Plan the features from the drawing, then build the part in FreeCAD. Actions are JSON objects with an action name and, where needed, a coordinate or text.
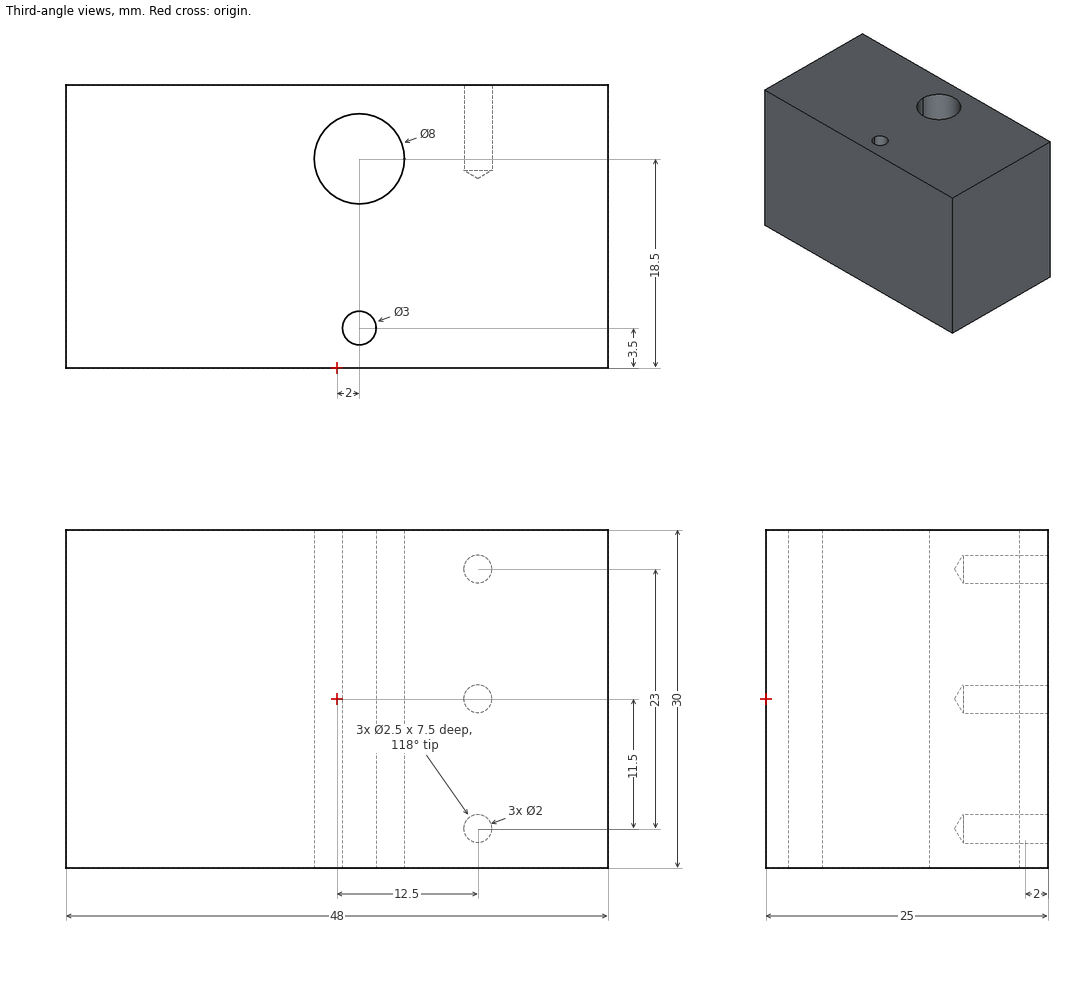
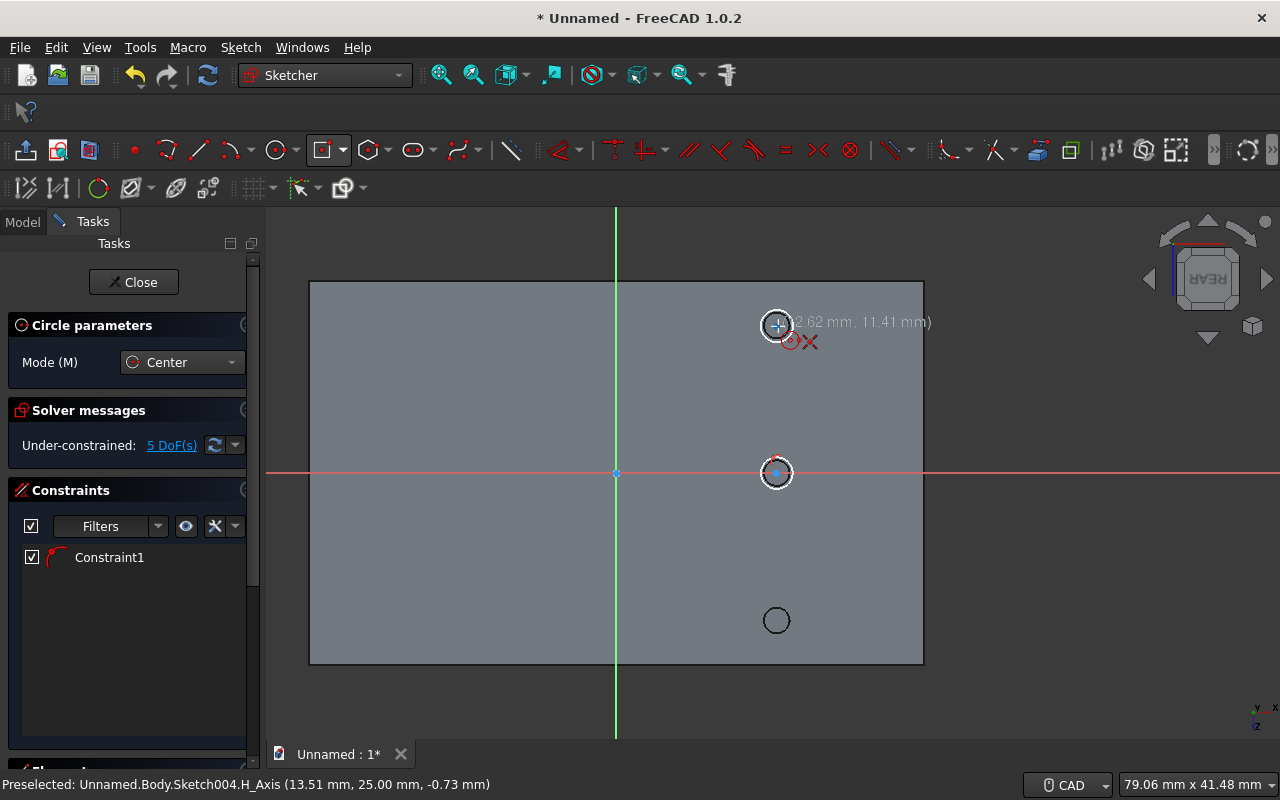
{"action": "scroll", "coordinate": [777, 621], "scroll_direction": "up", "scroll_amount": 2}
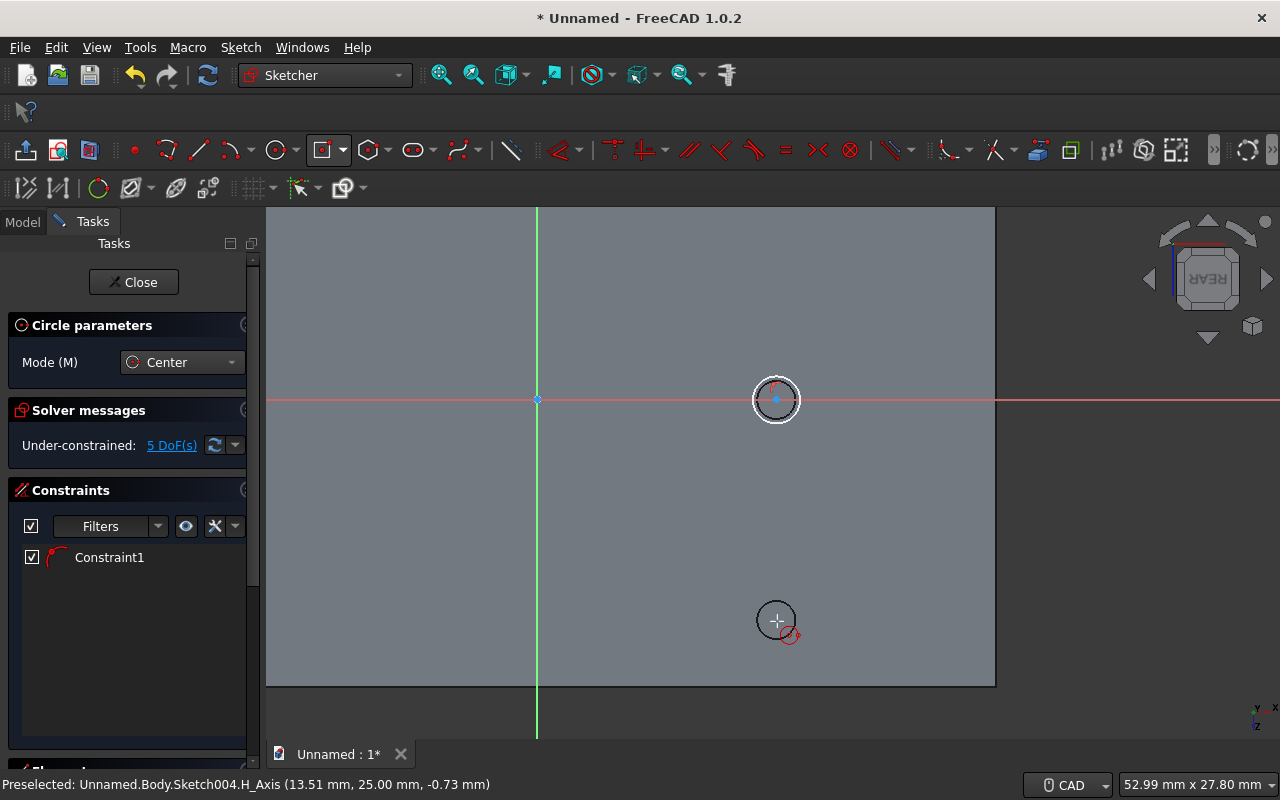
{"action": "left_click", "coordinate": [776, 620]}
{"action": "left_click", "coordinate": [793, 603]}
{"action": "key", "text": "Escape"}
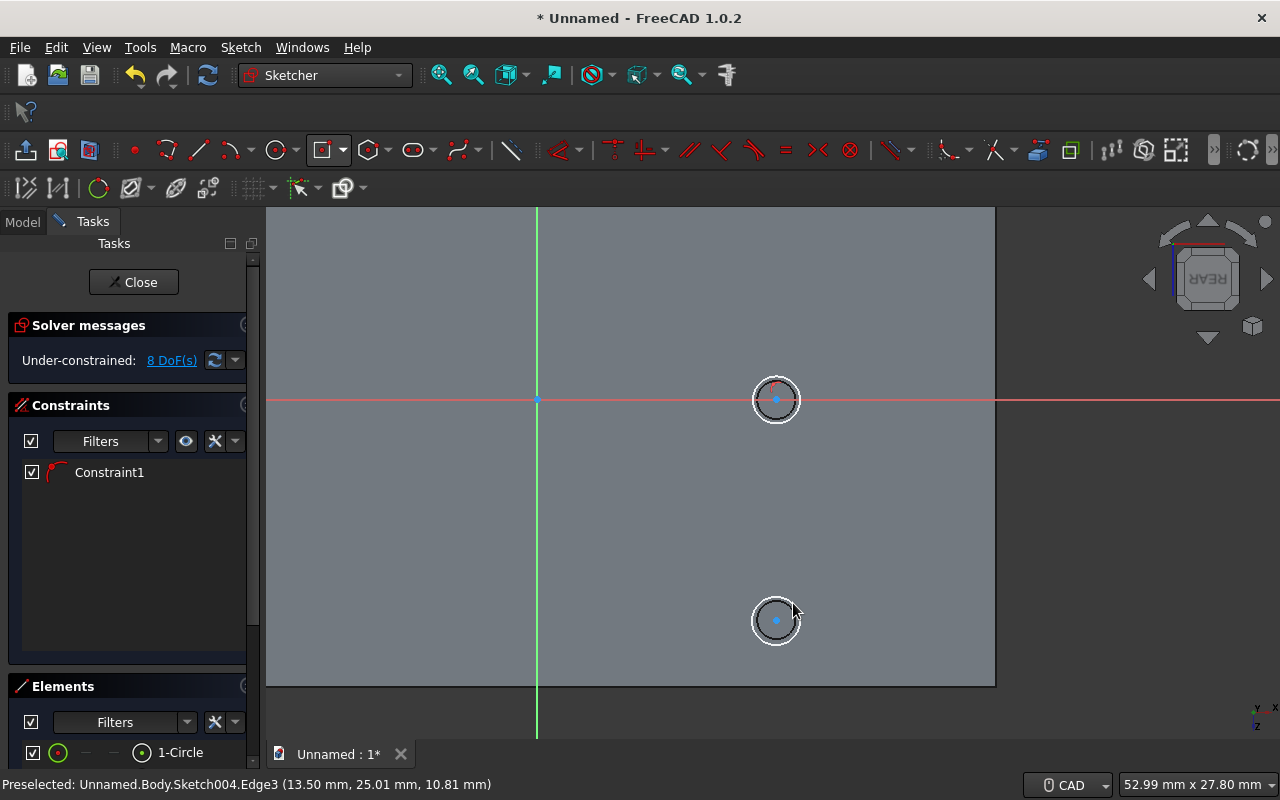
{"action": "scroll", "coordinate": [777, 622], "scroll_direction": "down", "scroll_amount": 2}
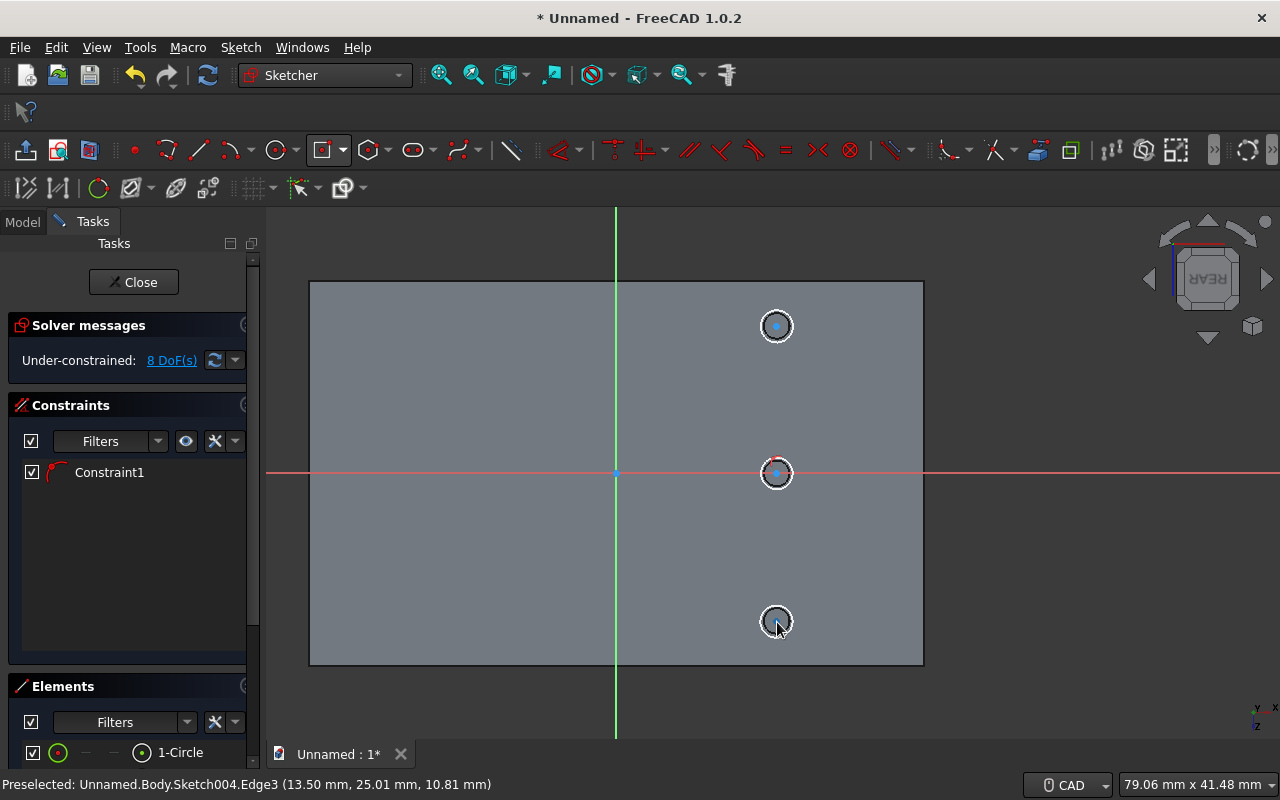
{"action": "left_click", "coordinate": [788, 315]}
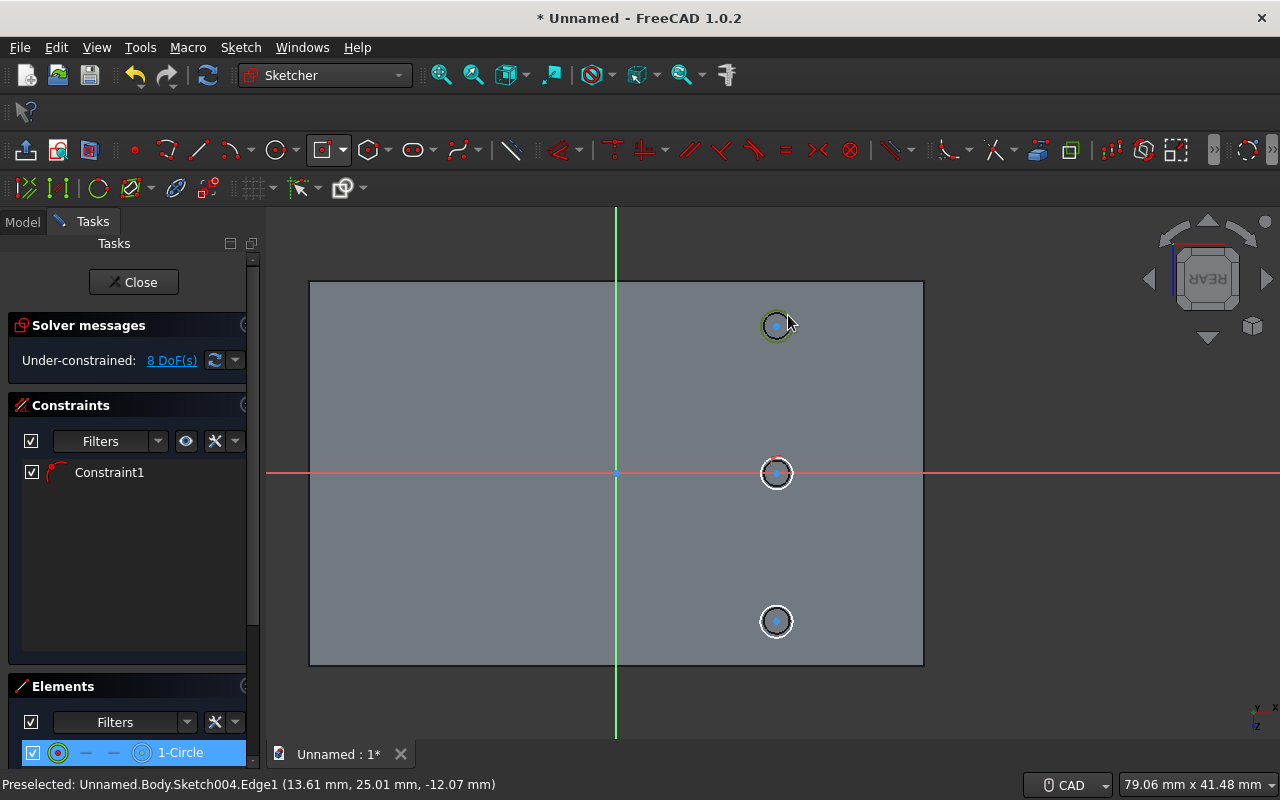
{"action": "scroll", "coordinate": [788, 462], "scroll_direction": "up", "scroll_amount": 2}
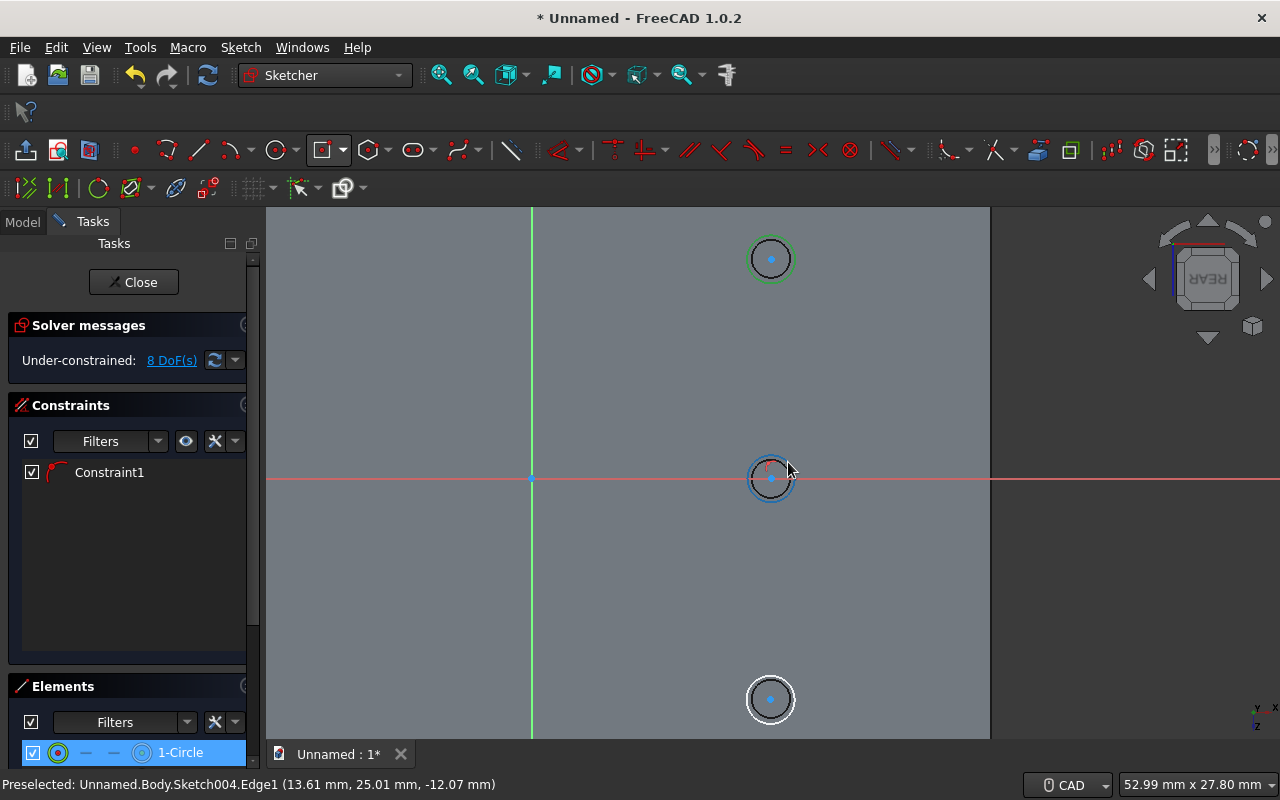
{"action": "left_click", "coordinate": [788, 462]}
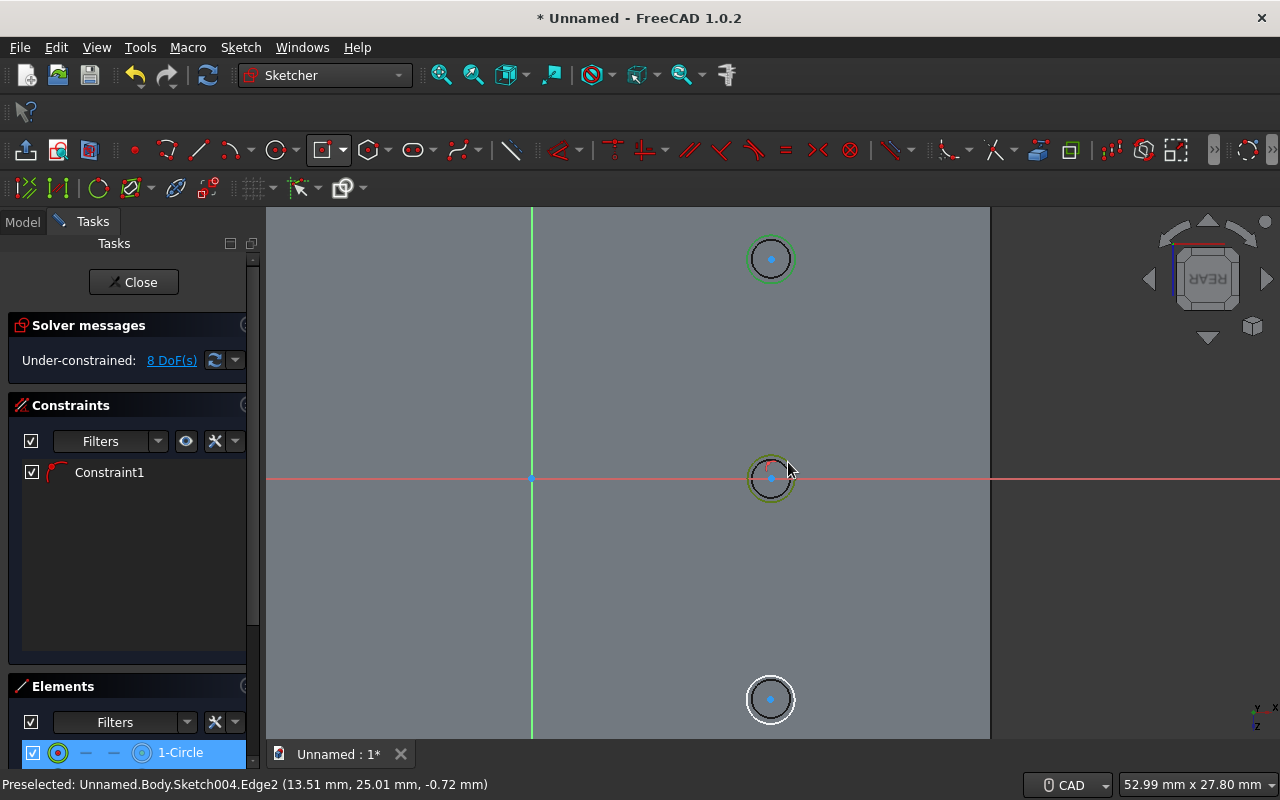
{"action": "left_click", "coordinate": [788, 683]}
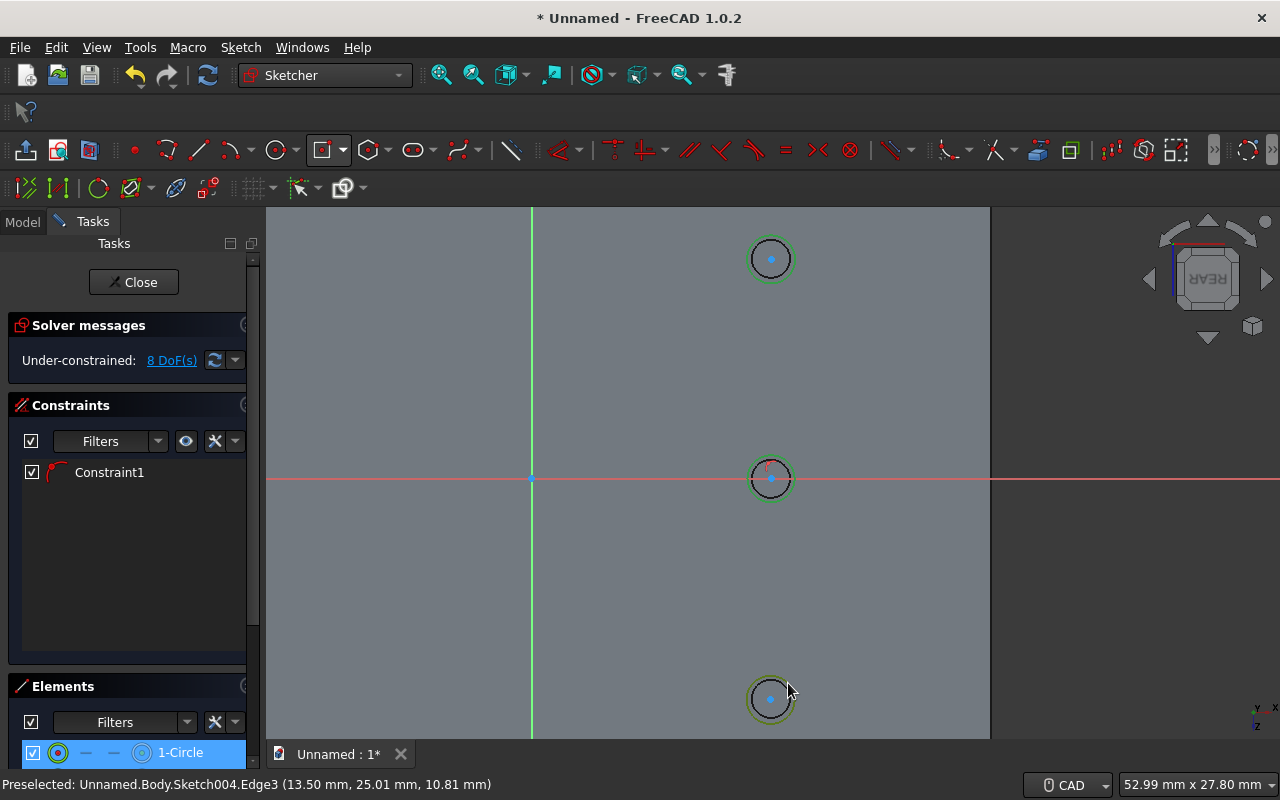
{"action": "left_click", "coordinate": [786, 150]}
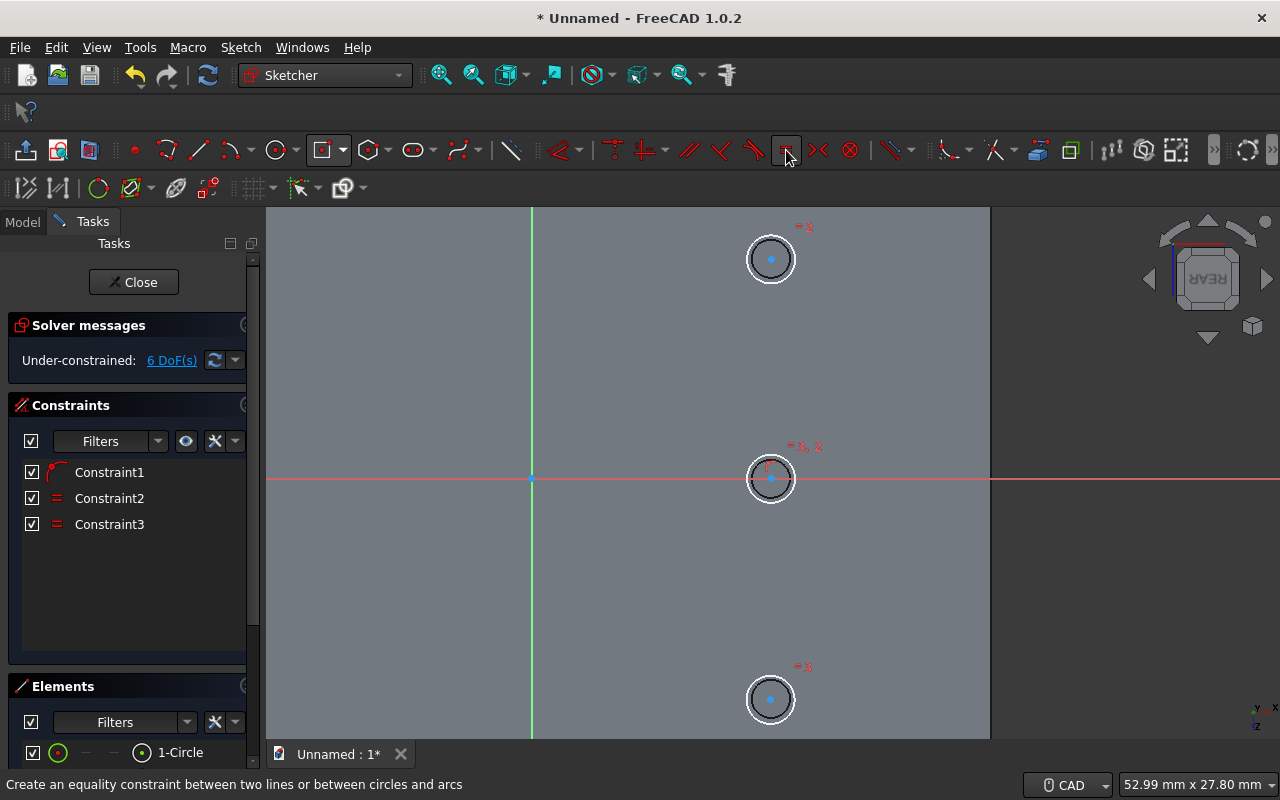
{"action": "left_click", "coordinate": [771, 259]}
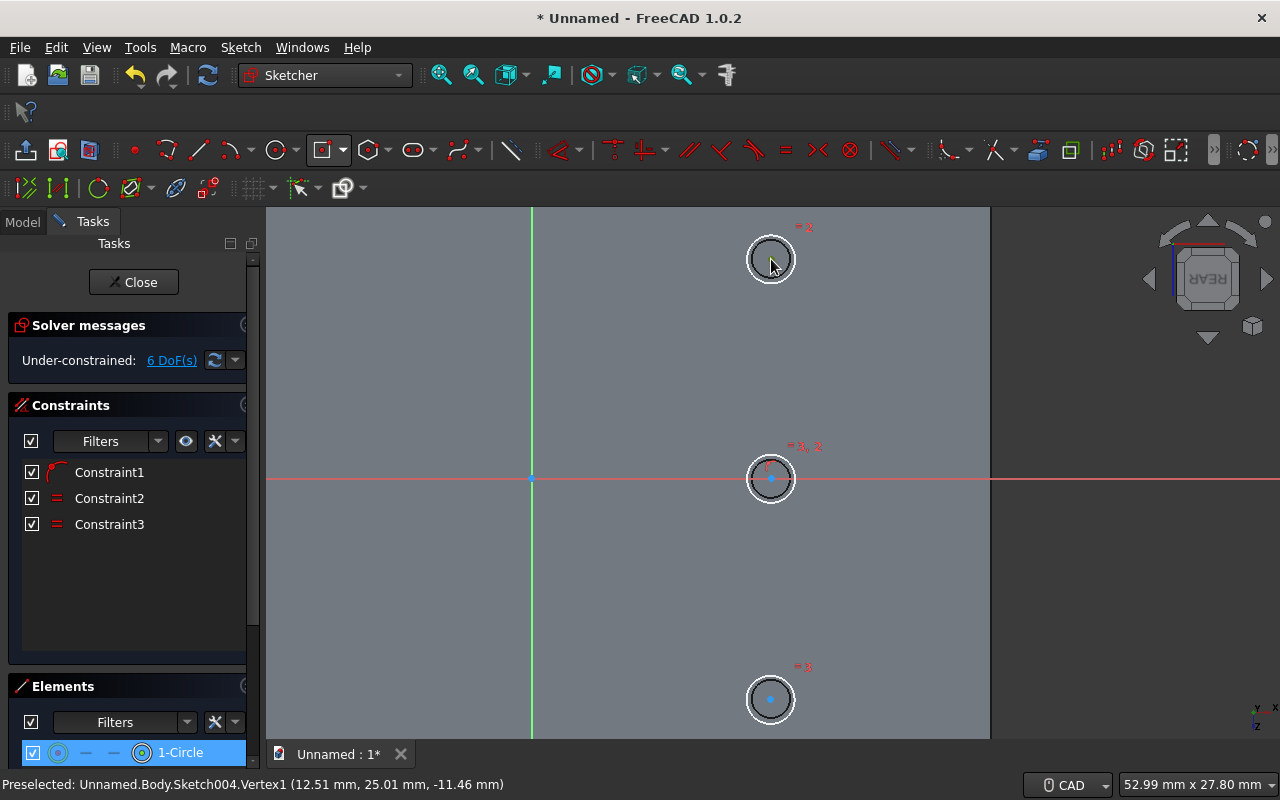
{"action": "left_click", "coordinate": [771, 479]}